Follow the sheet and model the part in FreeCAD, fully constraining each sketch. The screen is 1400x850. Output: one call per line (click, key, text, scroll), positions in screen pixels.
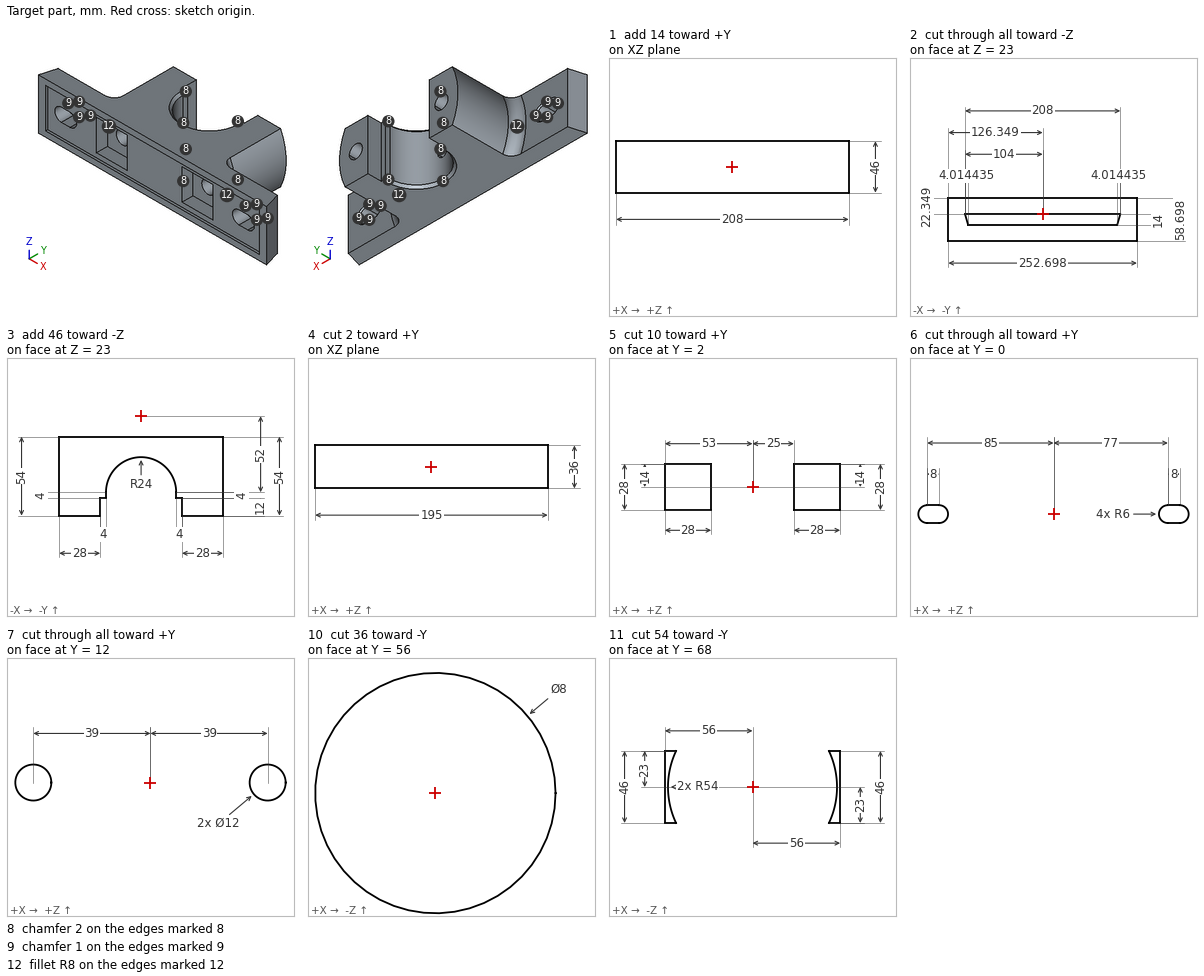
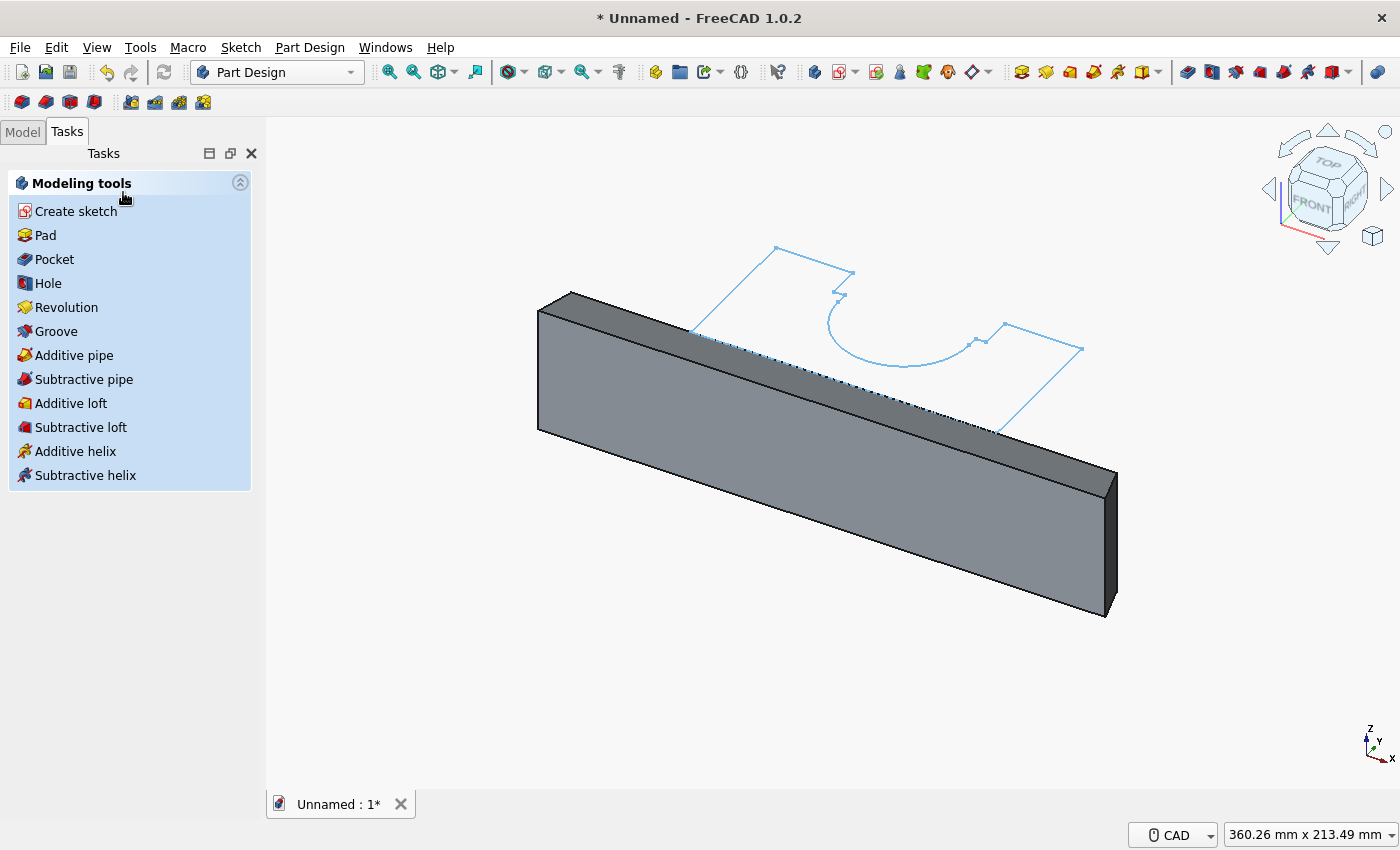
click(1022, 72)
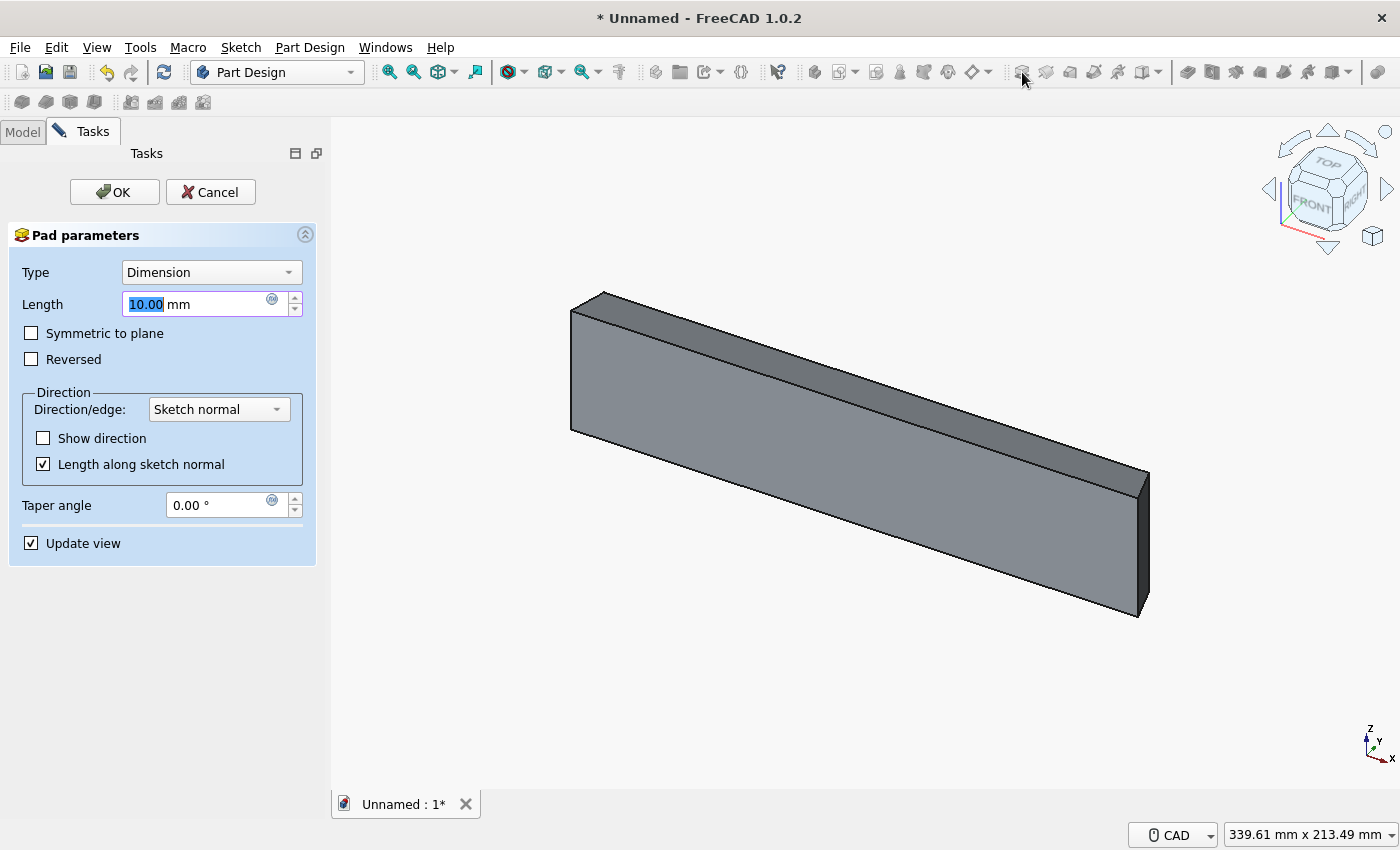
text(46)
key(Tab)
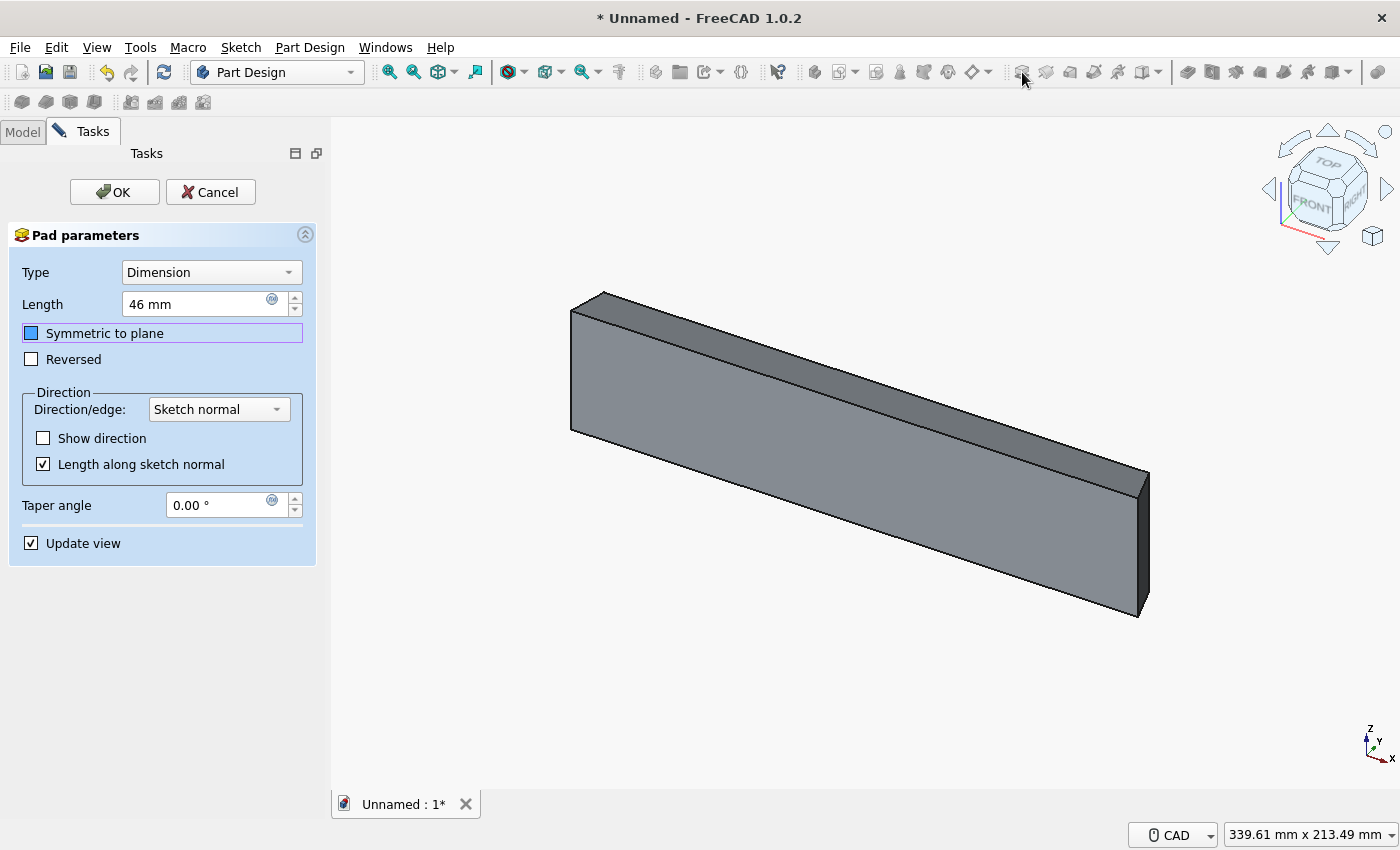
click(30, 359)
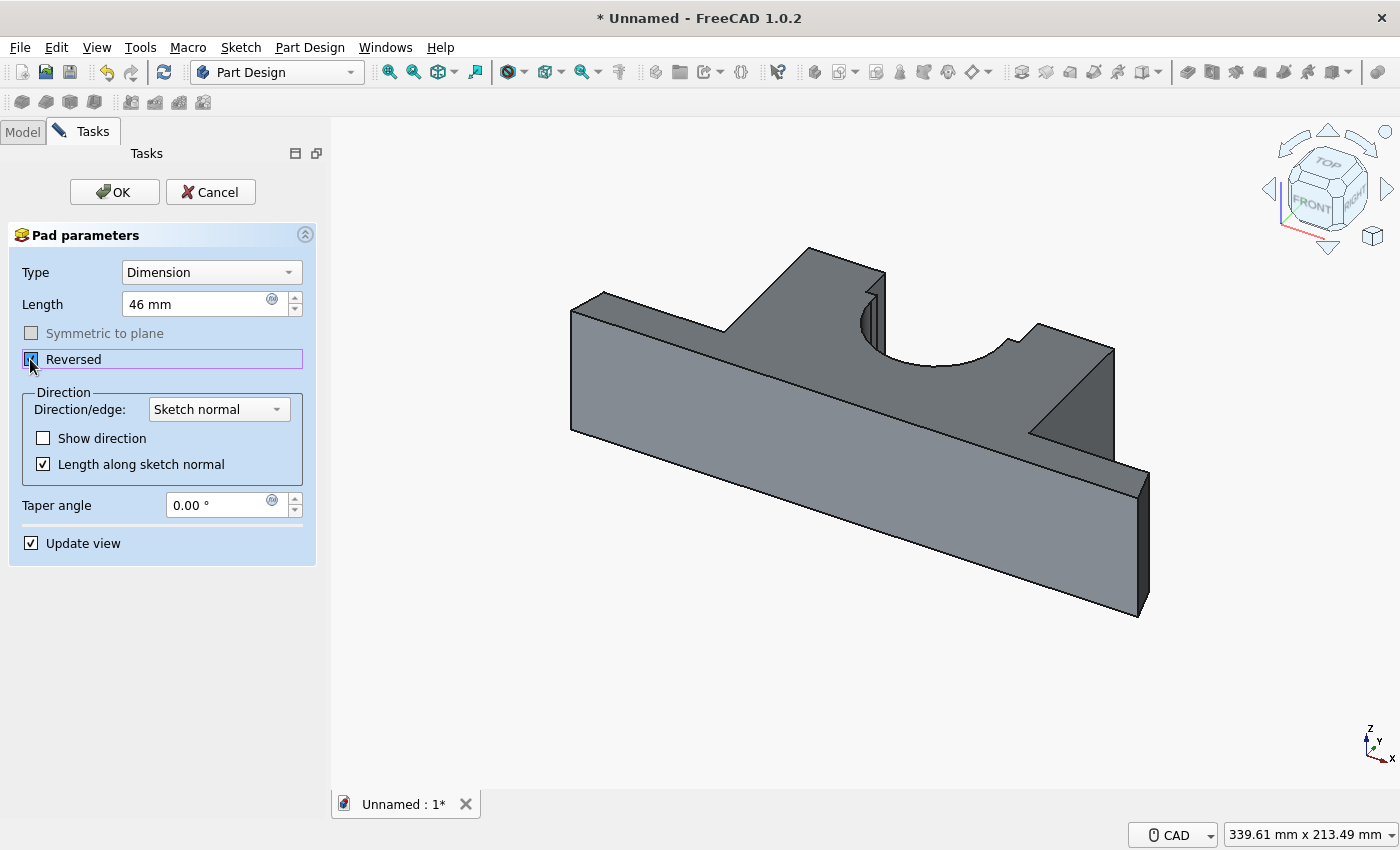
click(115, 192)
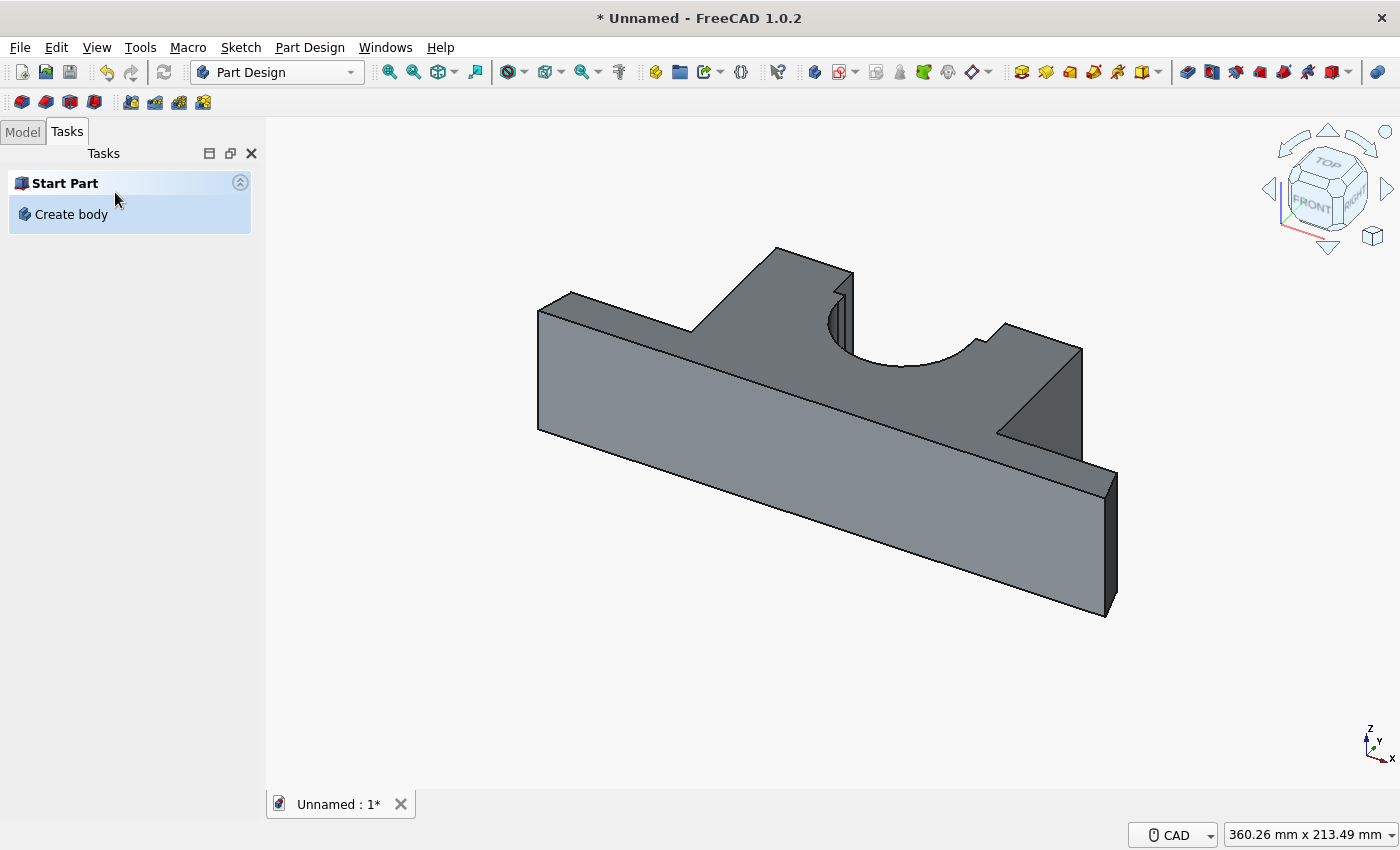
click(840, 72)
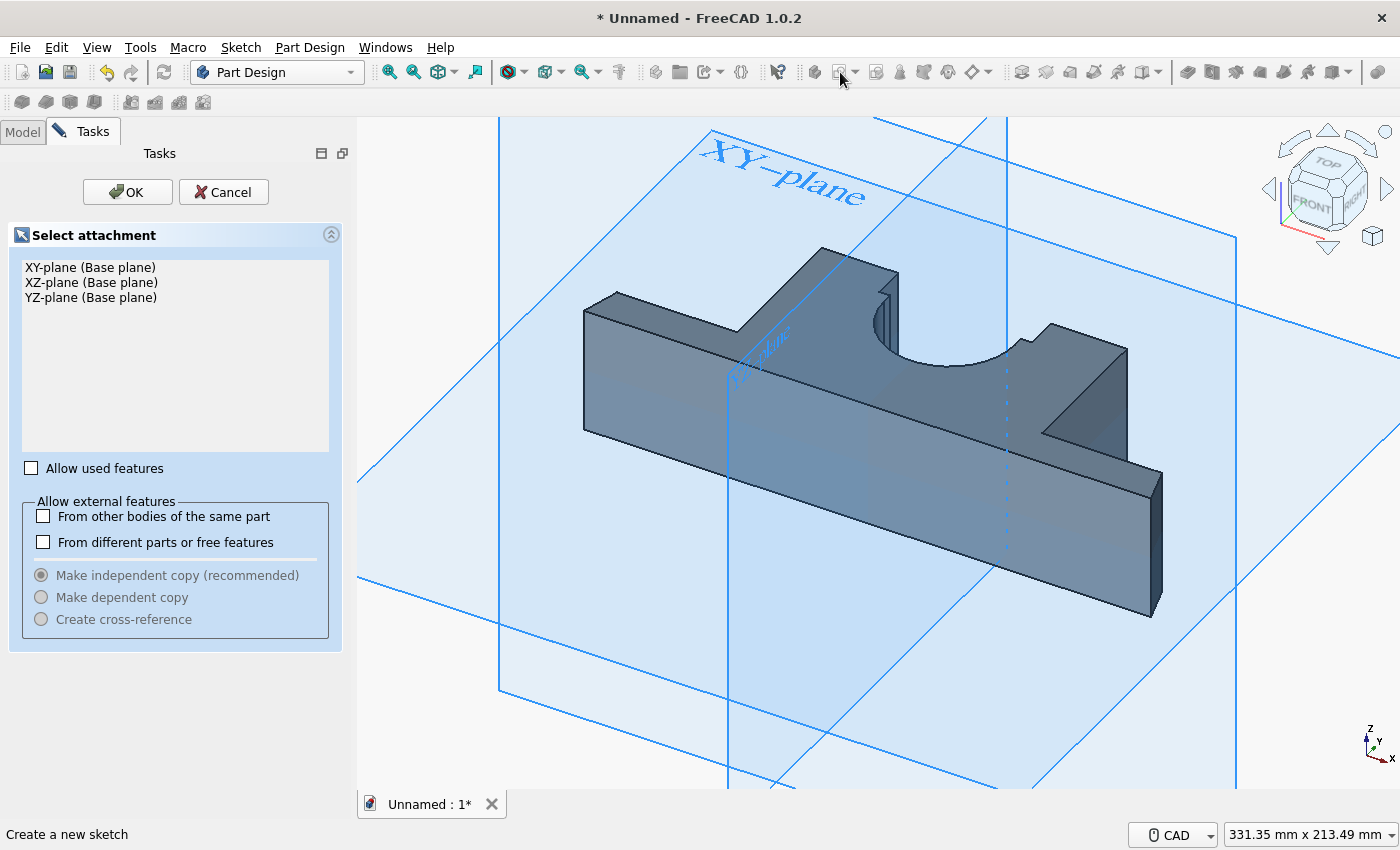
click(82, 282)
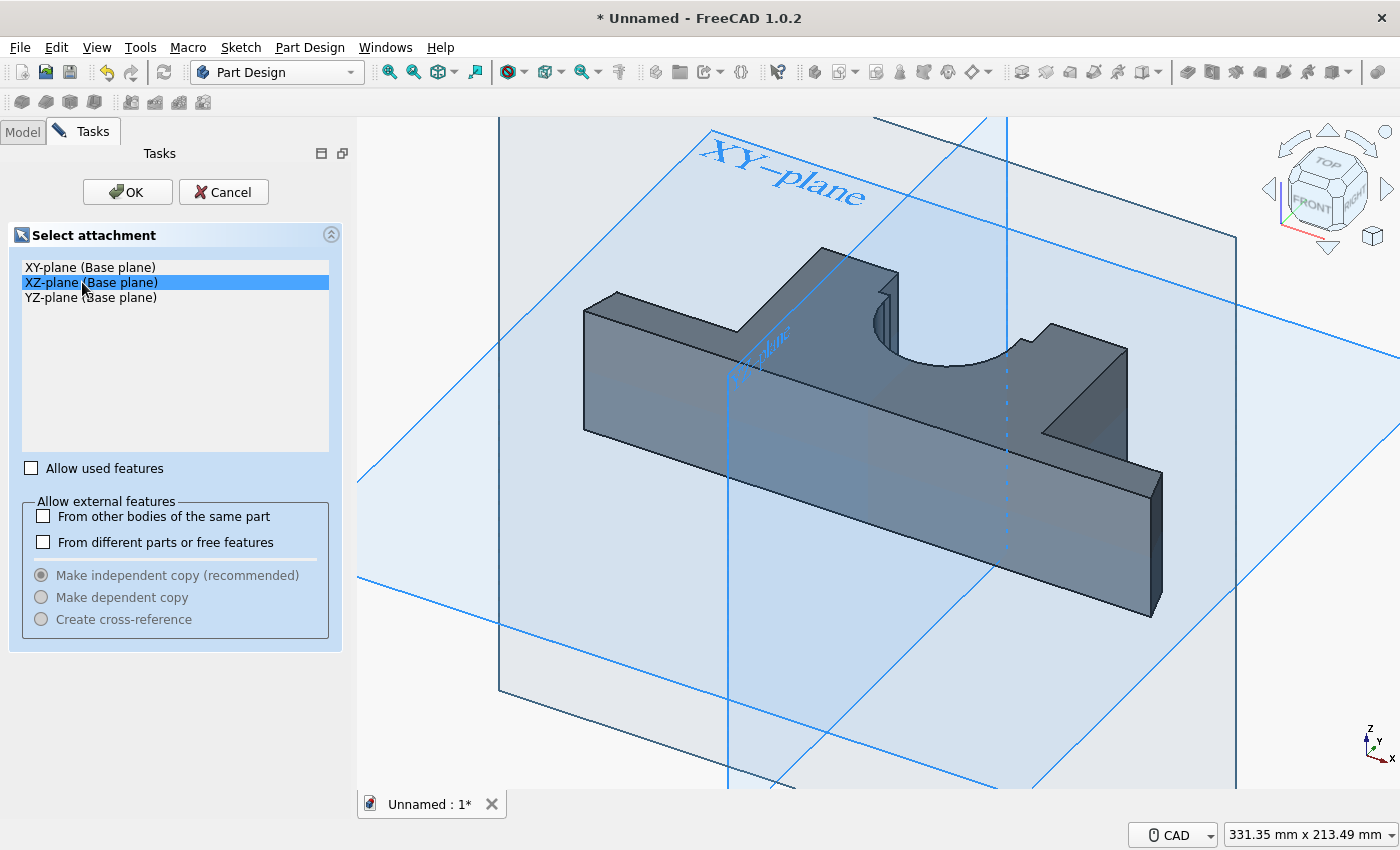
click(128, 192)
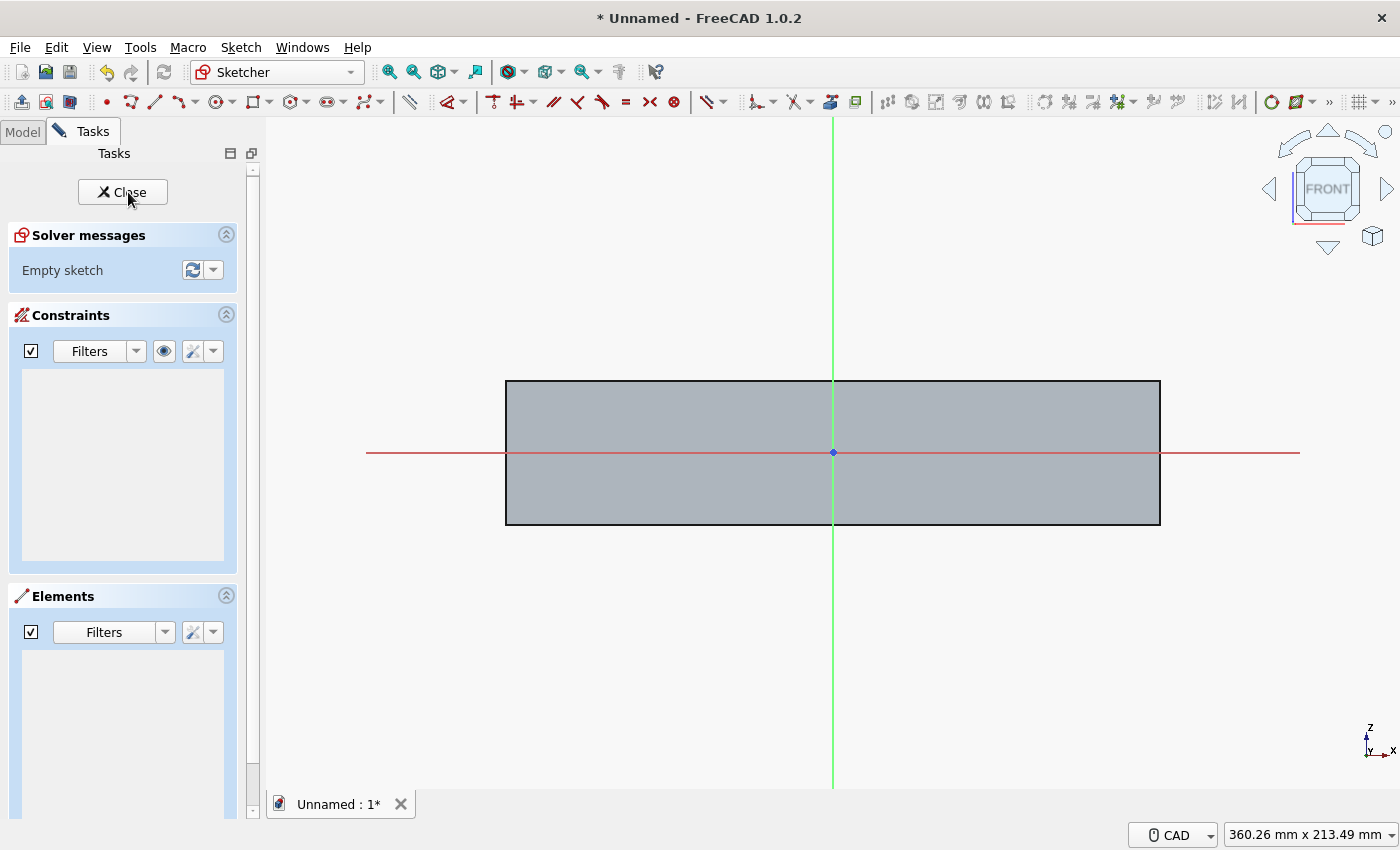
key(g)
key(v)